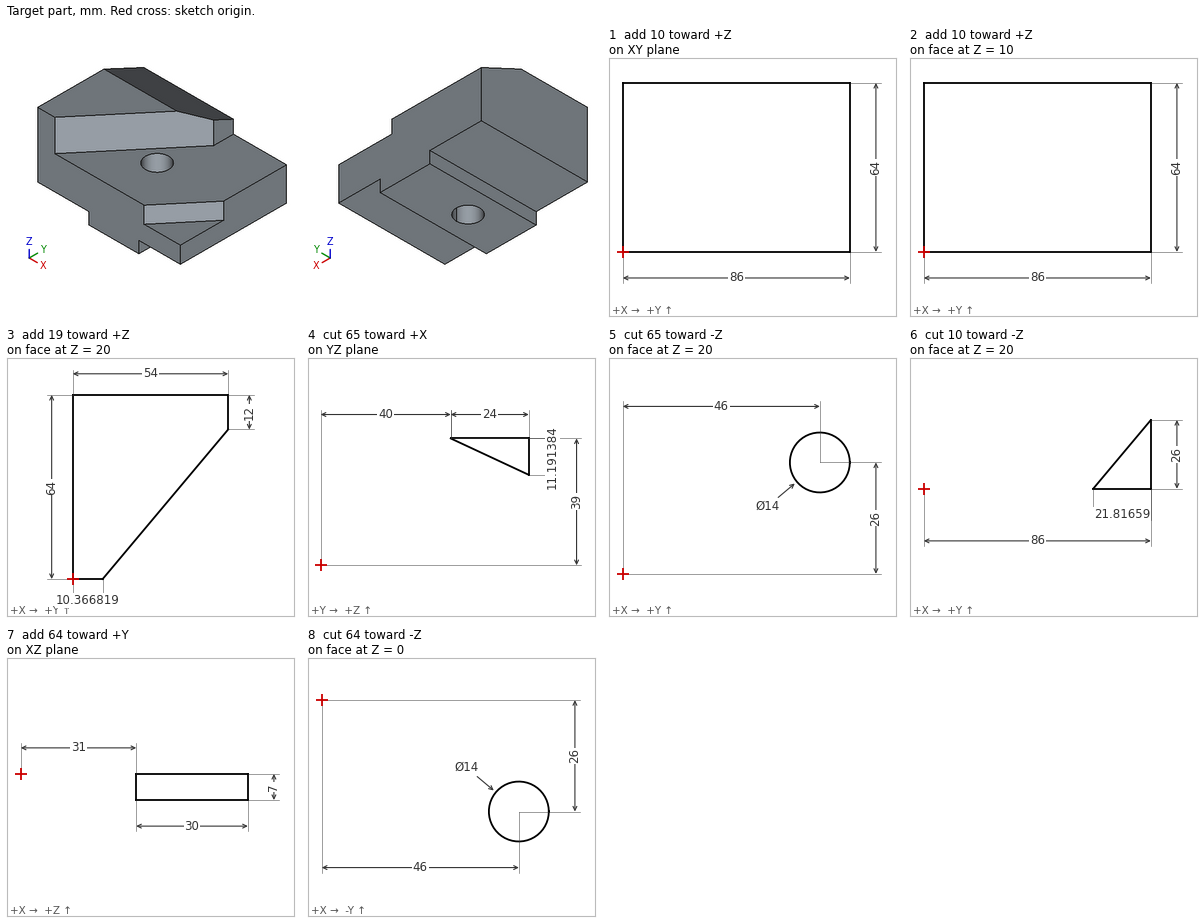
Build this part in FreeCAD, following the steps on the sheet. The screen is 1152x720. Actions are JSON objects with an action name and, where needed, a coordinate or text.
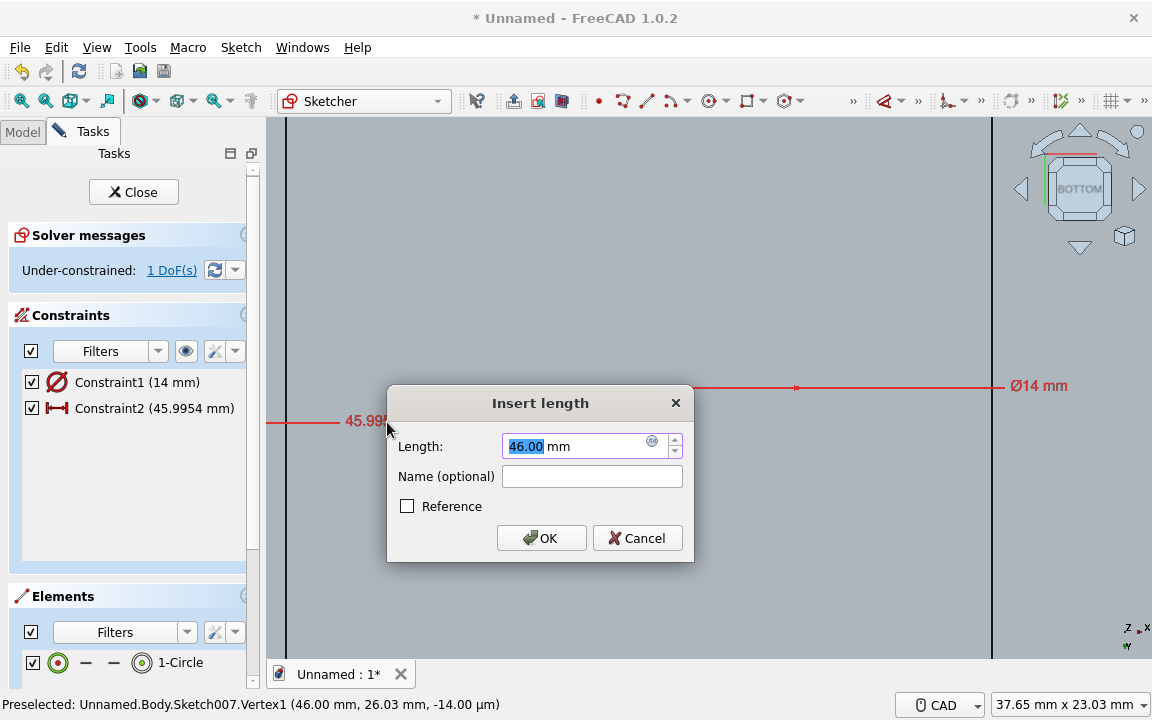
{"action": "type", "text": "46"}
{"action": "key", "text": "Return"}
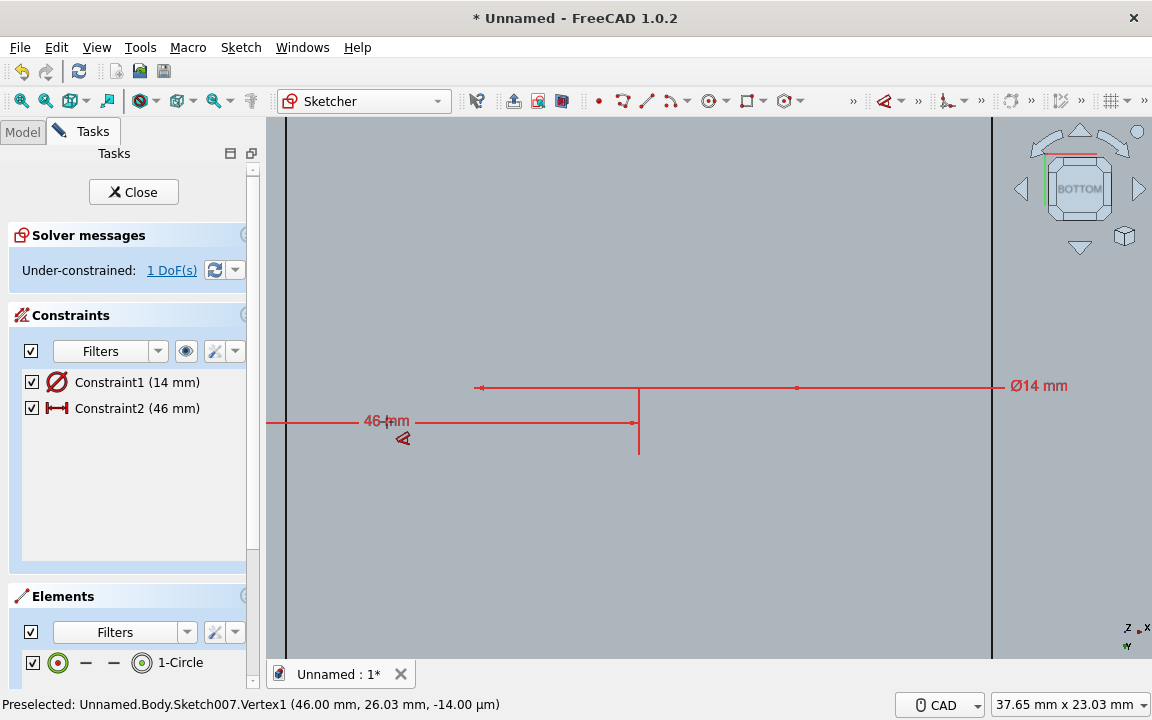
{"action": "left_click", "coordinate": [639, 388]}
{"action": "left_click", "coordinate": [673, 266]}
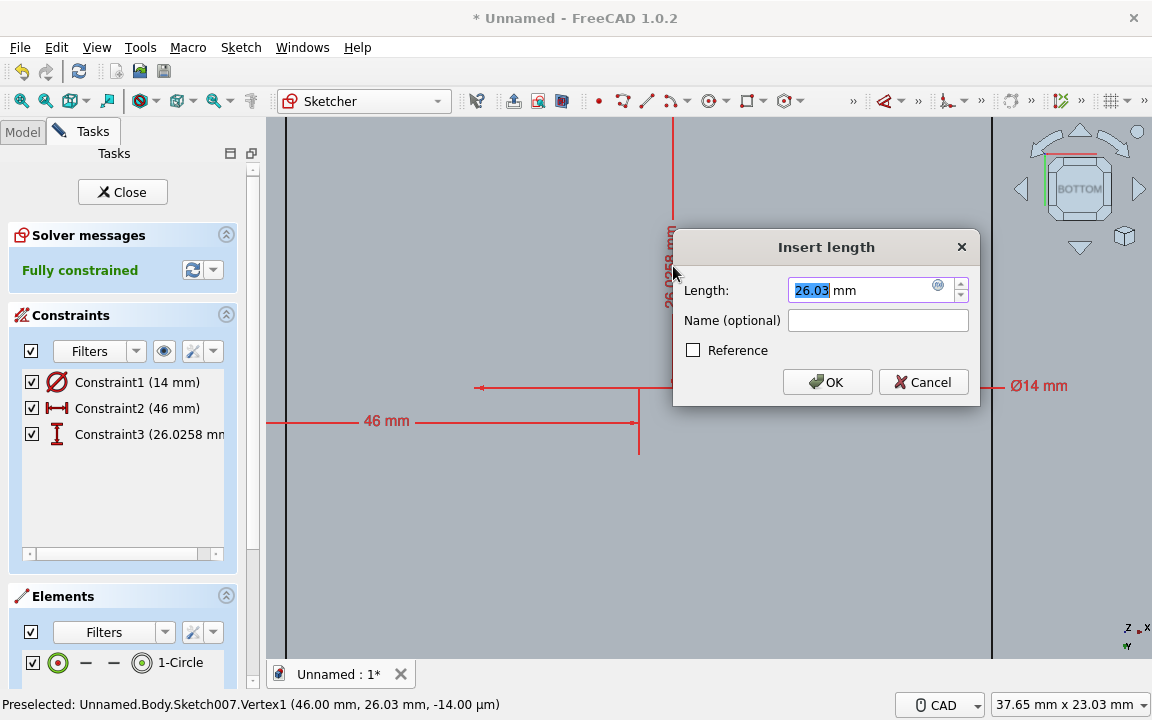
{"action": "type", "text": "26"}
{"action": "key", "text": "Return"}
{"action": "key", "text": "Escape"}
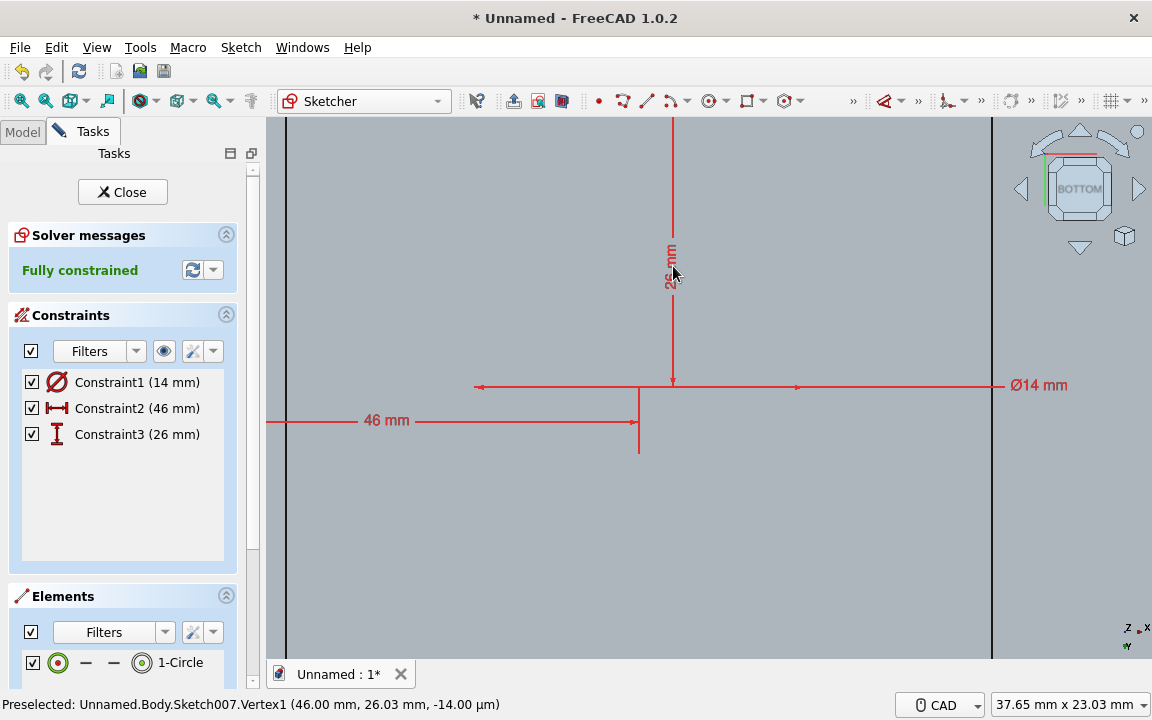
{"action": "left_click", "coordinate": [123, 192]}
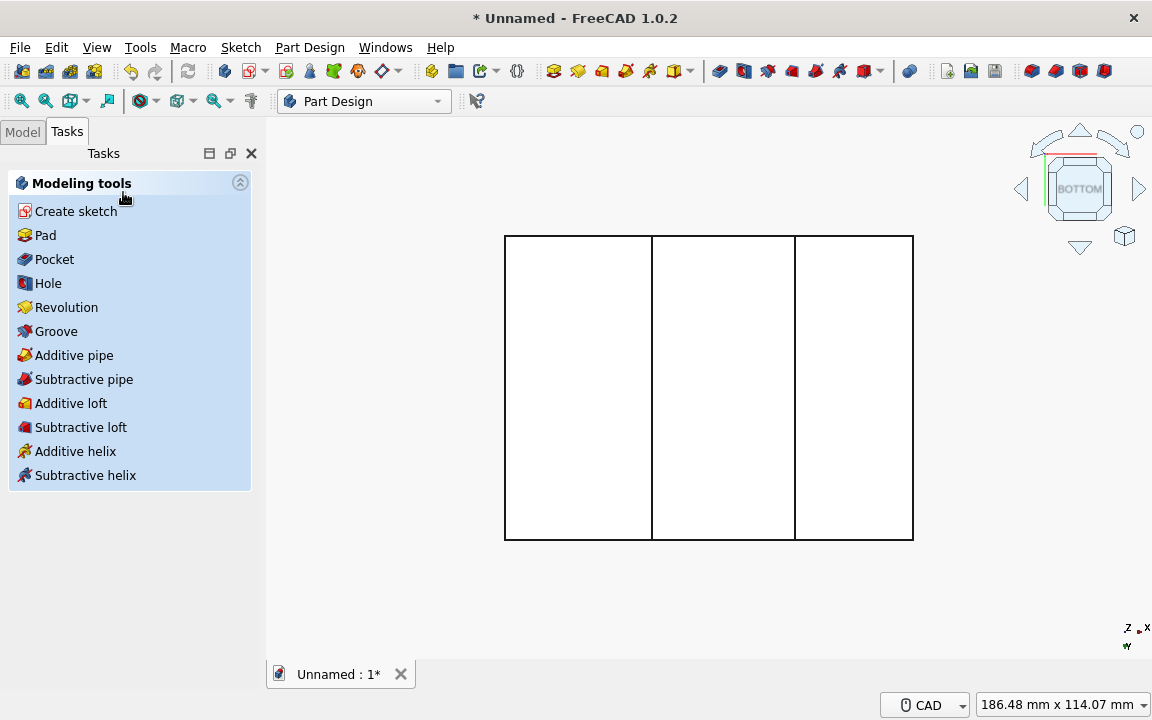
{"action": "left_click", "coordinate": [720, 72]}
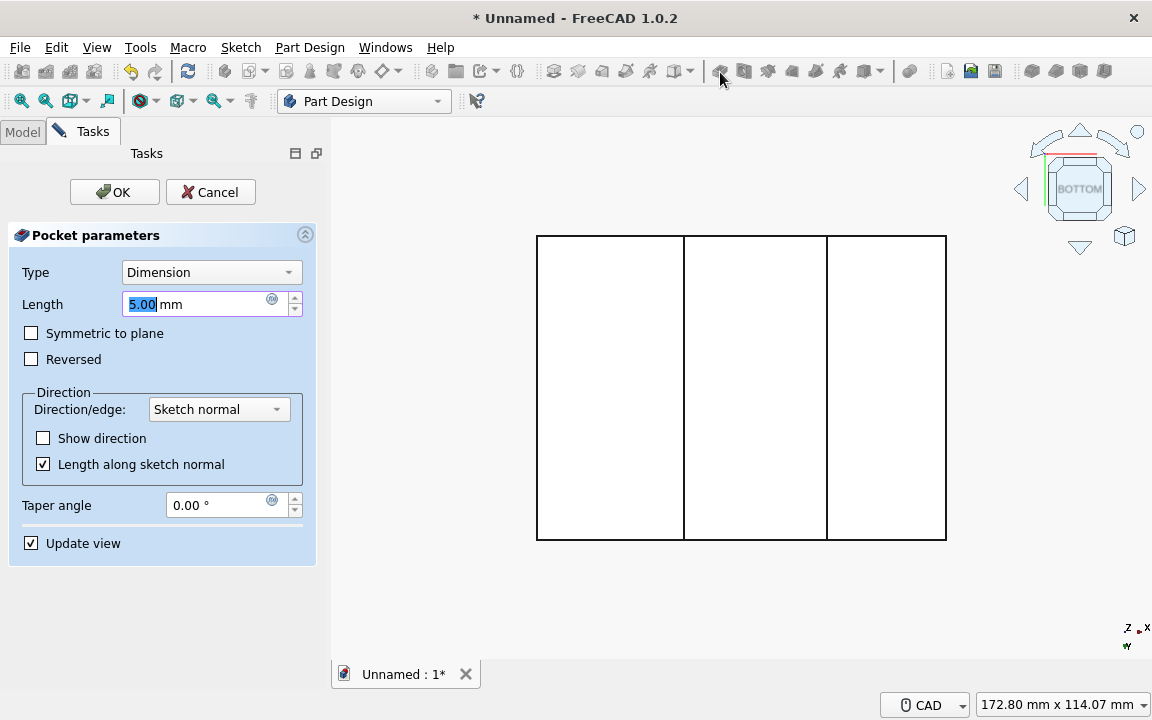
{"action": "type", "text": "64"}
{"action": "key", "text": "Tab"}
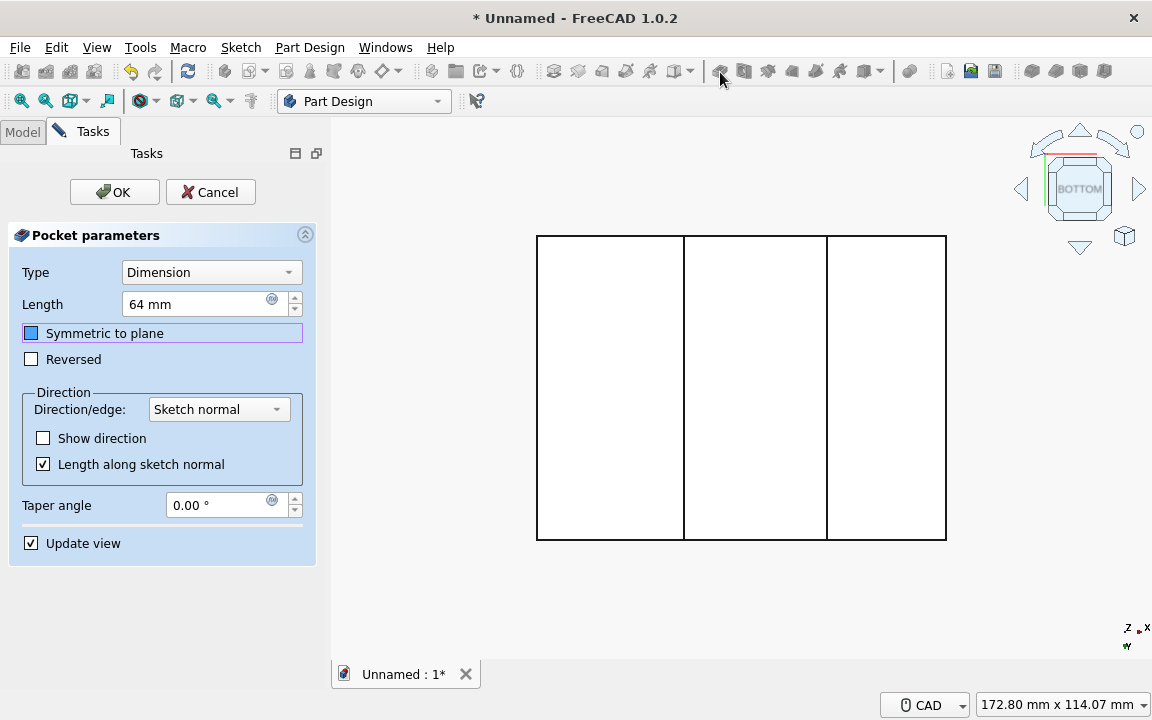
{"action": "left_click", "coordinate": [30, 359]}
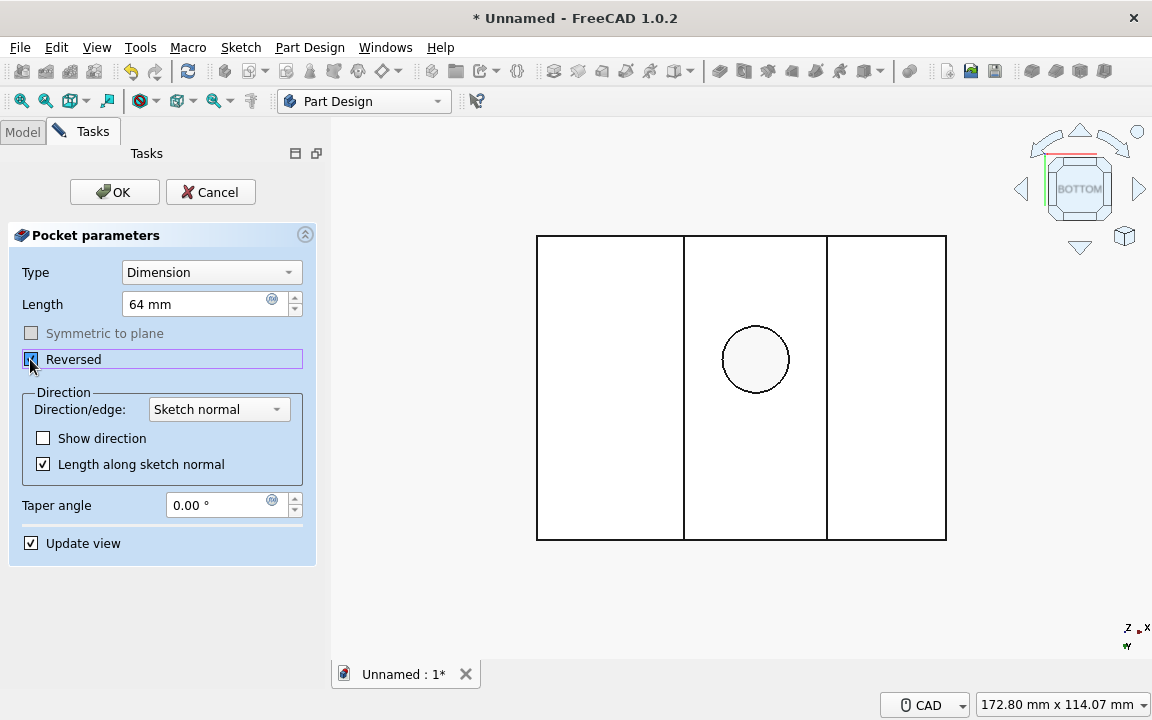
{"action": "left_click", "coordinate": [115, 192]}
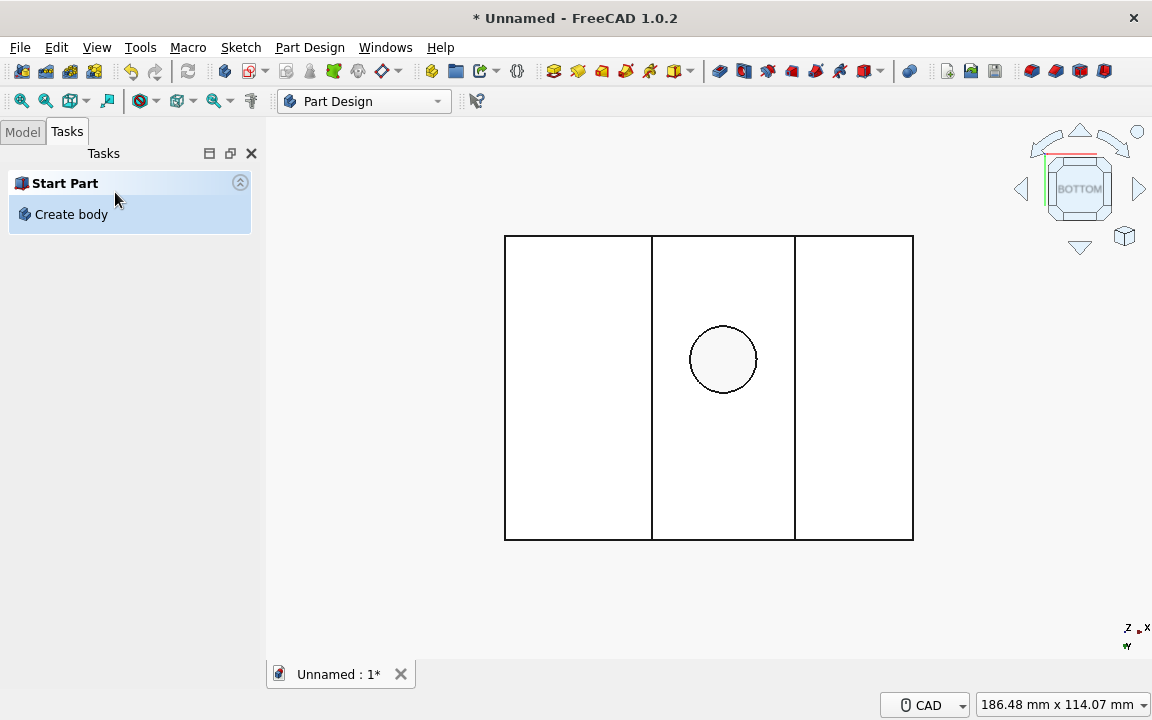
{"action": "key", "text": "0"}